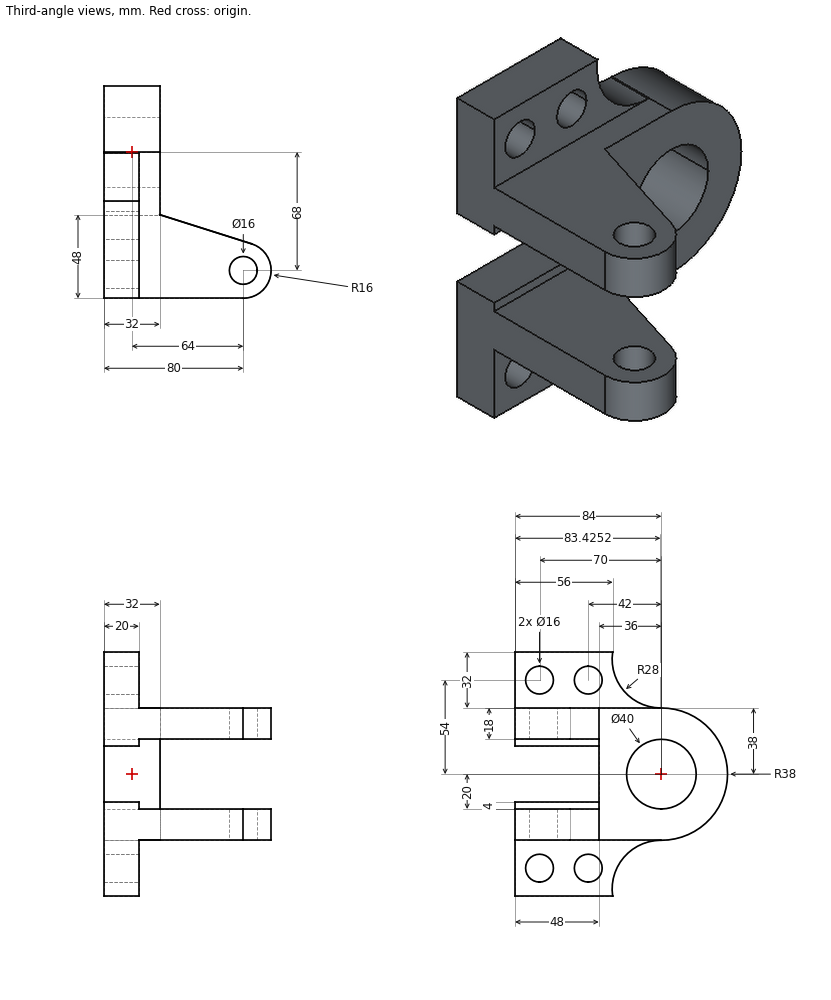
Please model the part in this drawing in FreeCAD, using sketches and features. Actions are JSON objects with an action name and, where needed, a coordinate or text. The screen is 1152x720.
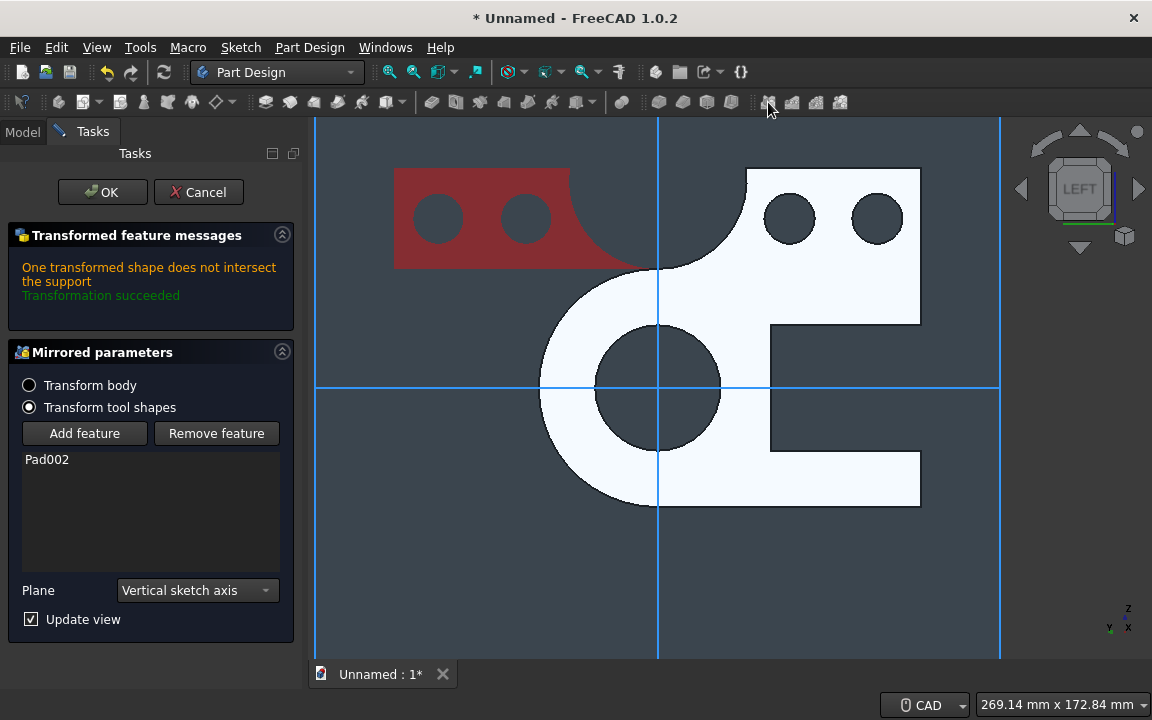
{"action": "left_click", "coordinate": [198, 590]}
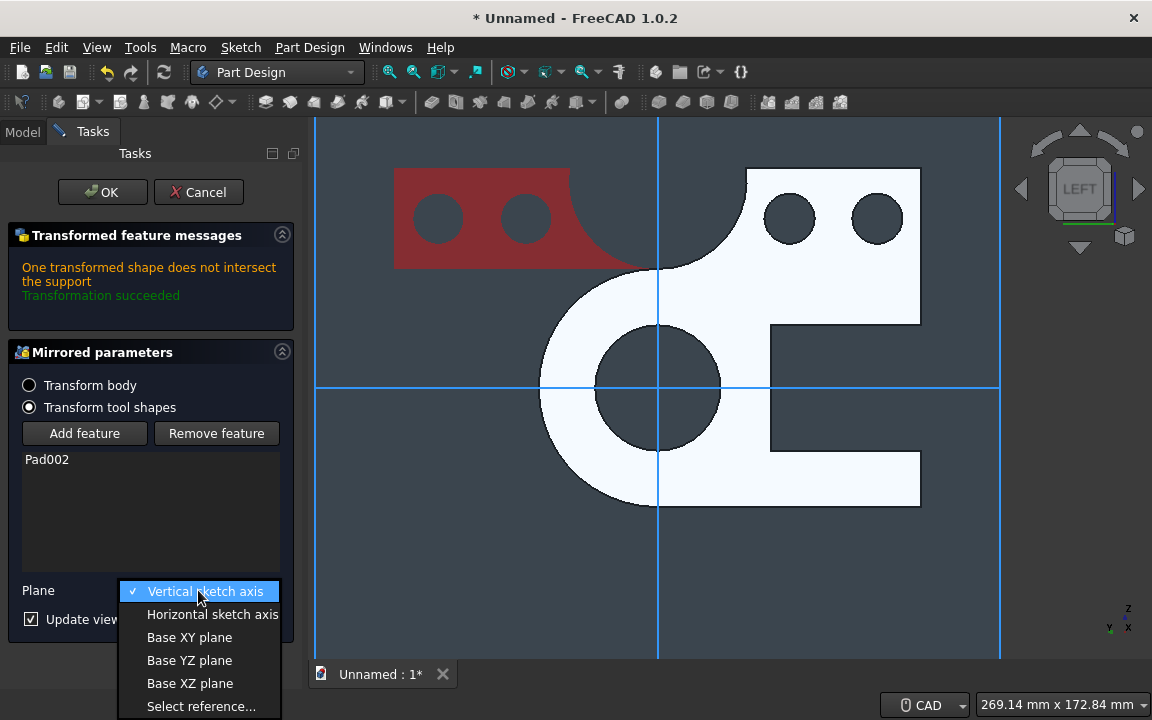
{"action": "left_click", "coordinate": [198, 638]}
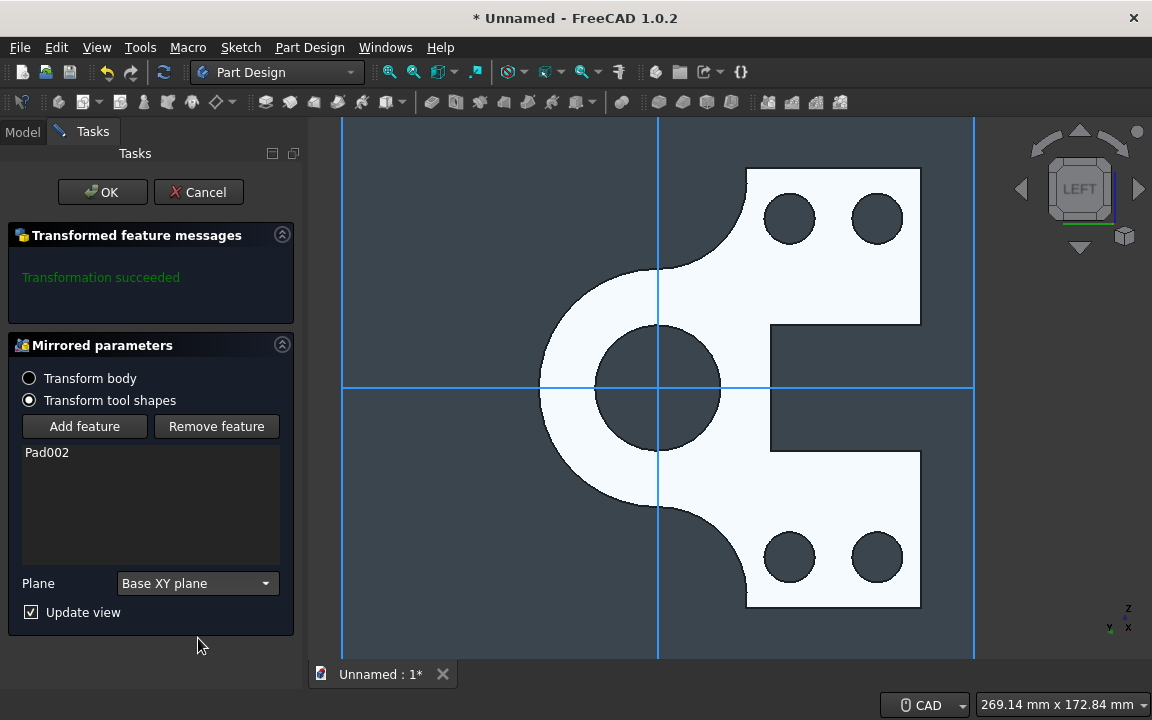
{"action": "left_click", "coordinate": [103, 192]}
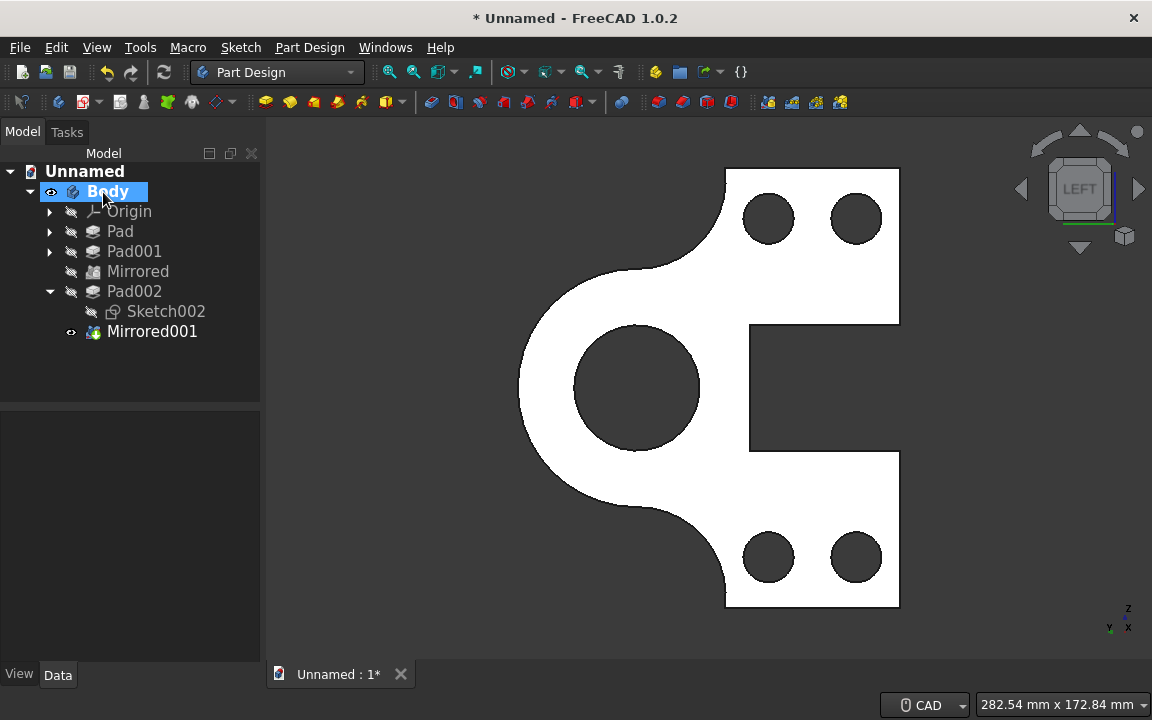
{"action": "left_click", "coordinate": [818, 512]}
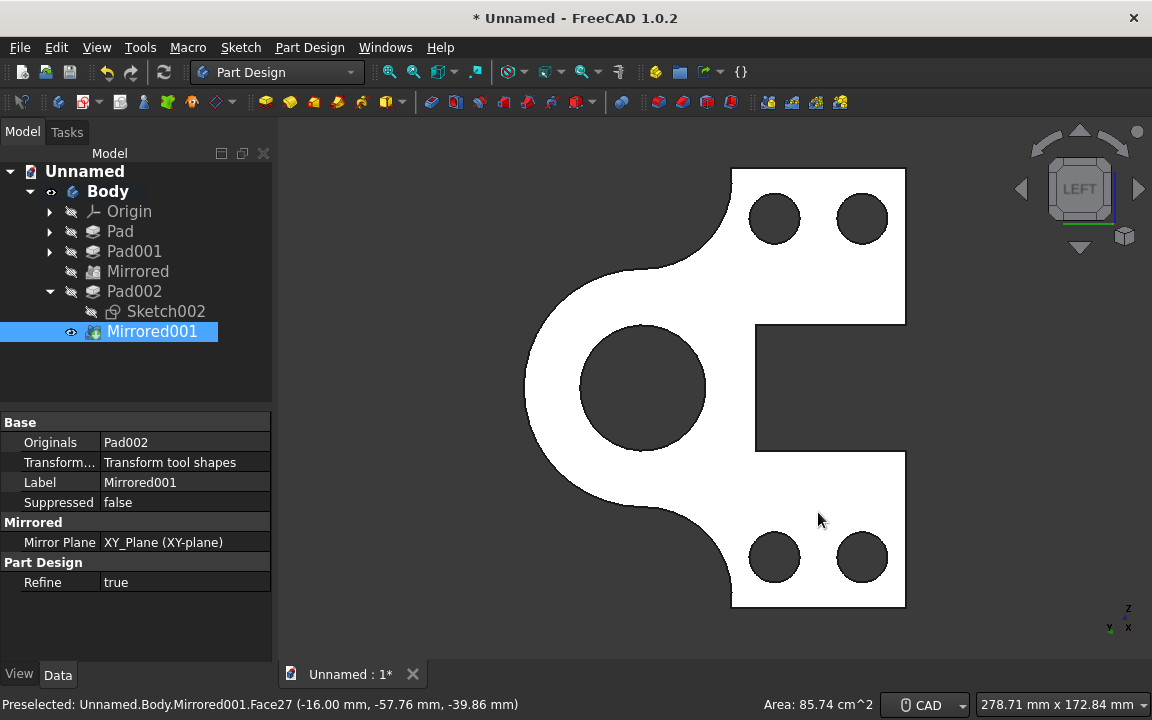
{"action": "left_click", "coordinate": [84, 102]}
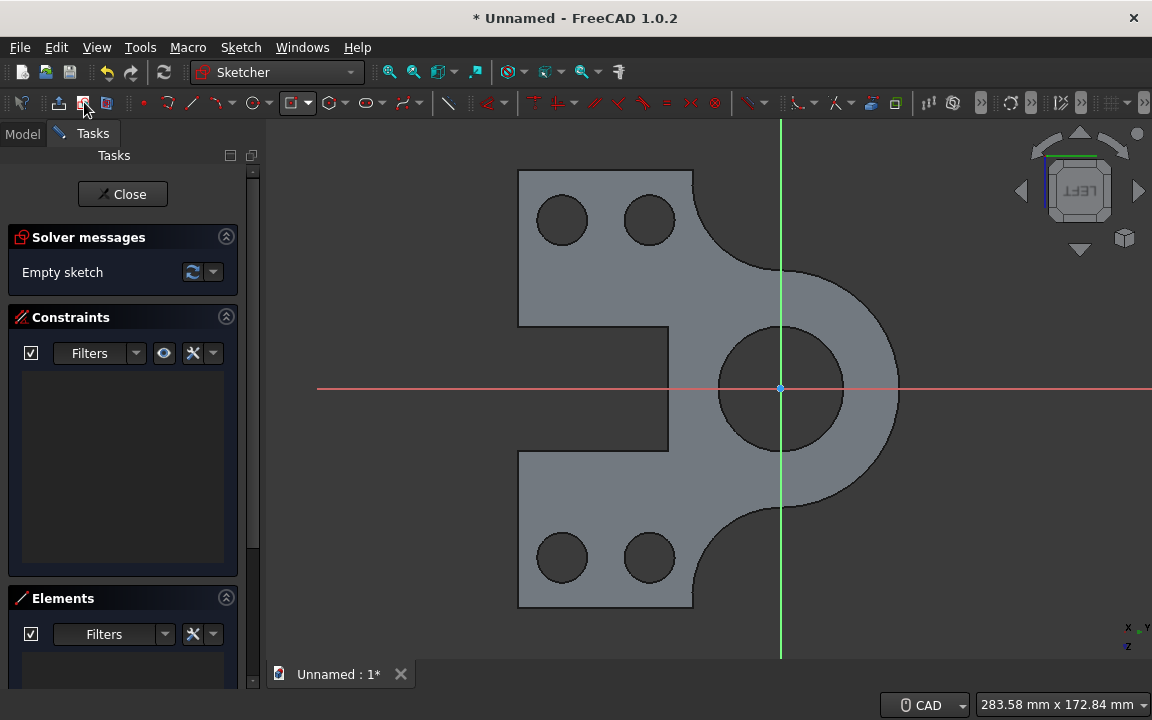
{"action": "scroll", "coordinate": [661, 320], "scroll_direction": "up", "scroll_amount": 3}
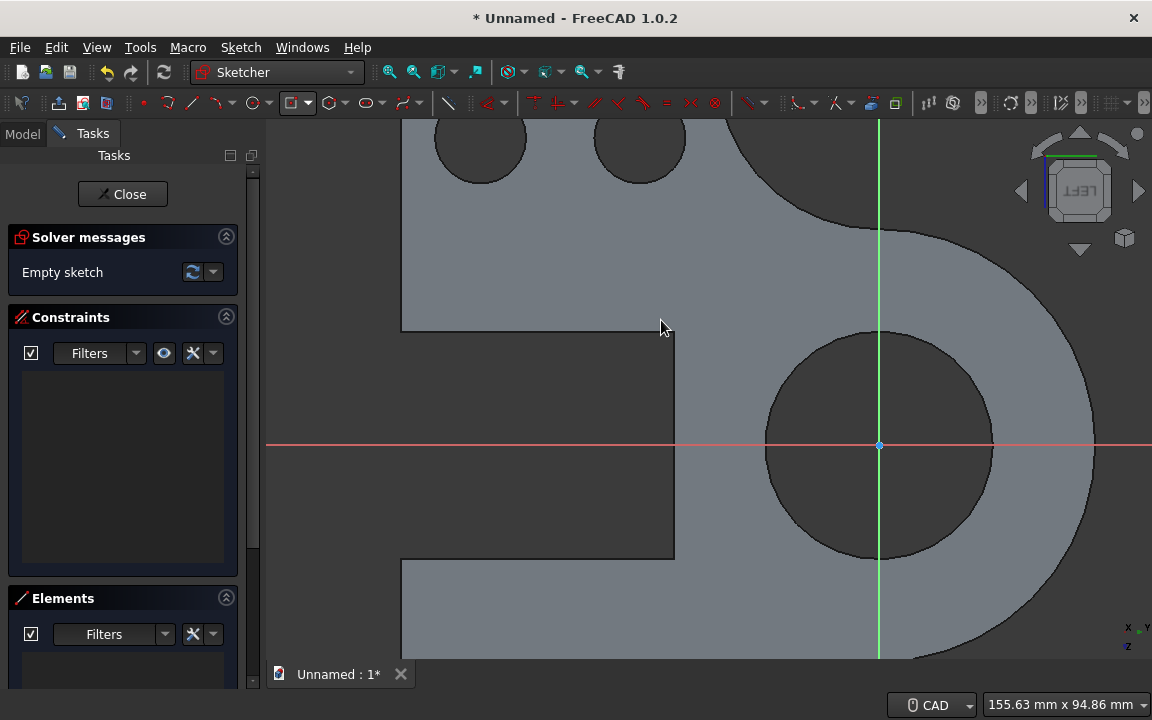
{"action": "key", "text": "g r"}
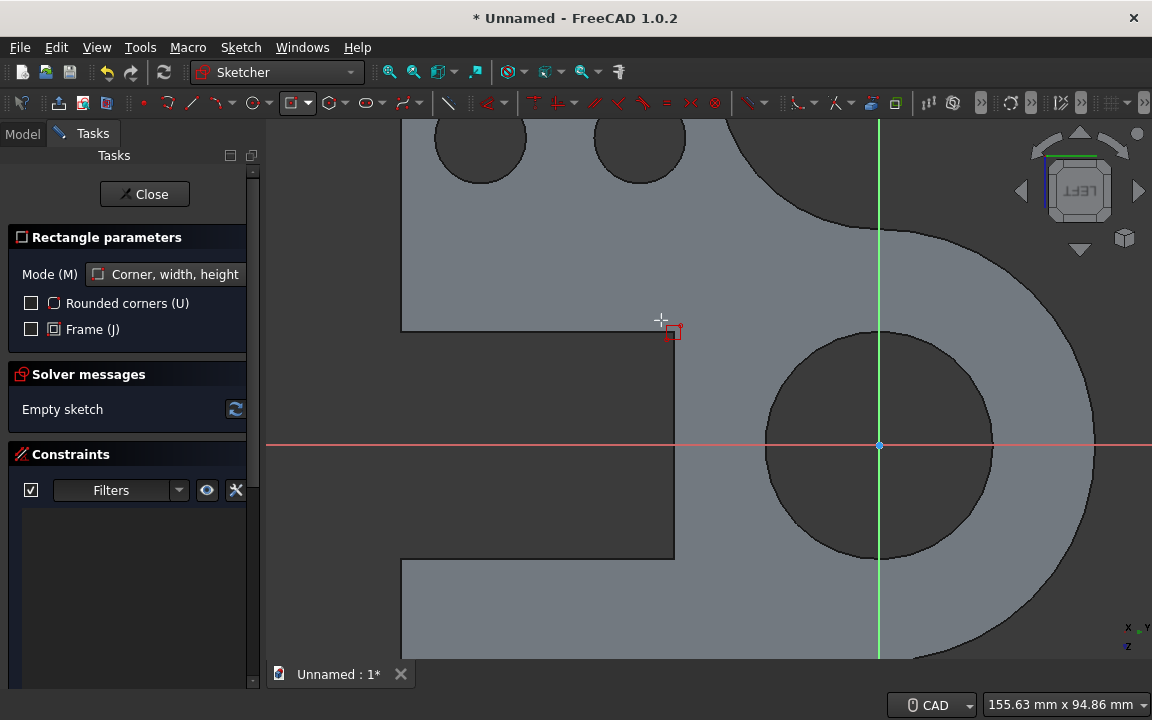
{"action": "left_click", "coordinate": [401, 332]}
{"action": "left_click", "coordinate": [674, 354]}
{"action": "key", "text": "Escape"}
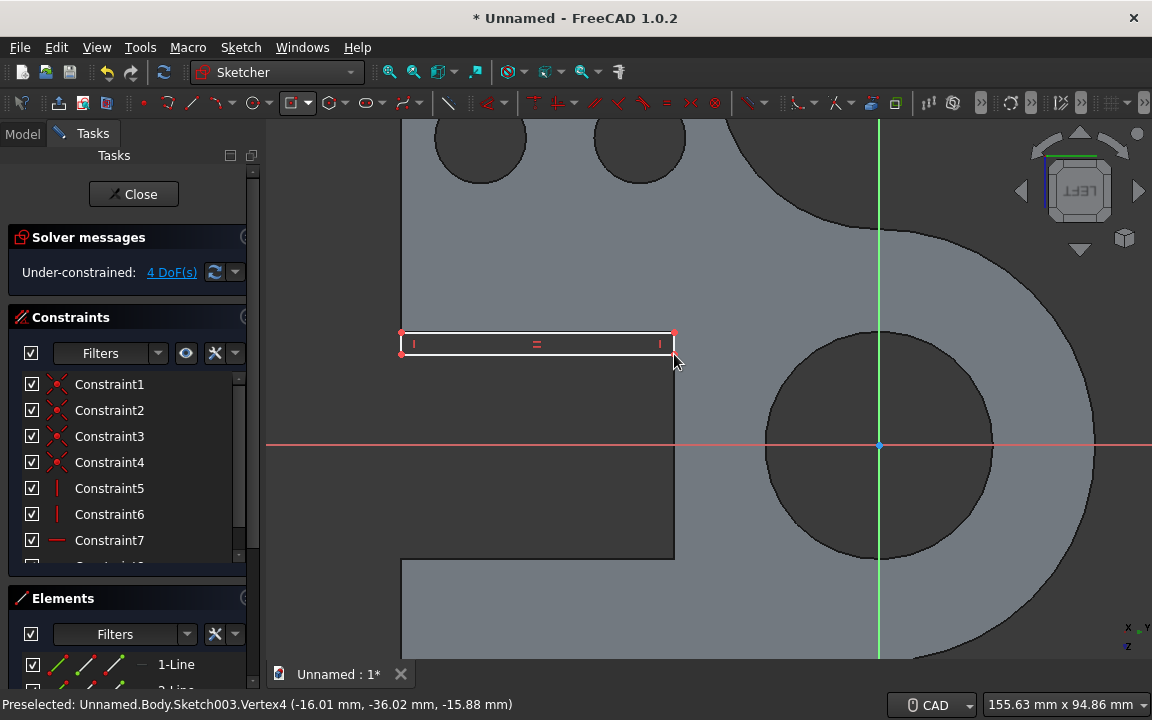
{"action": "left_click", "coordinate": [488, 104]}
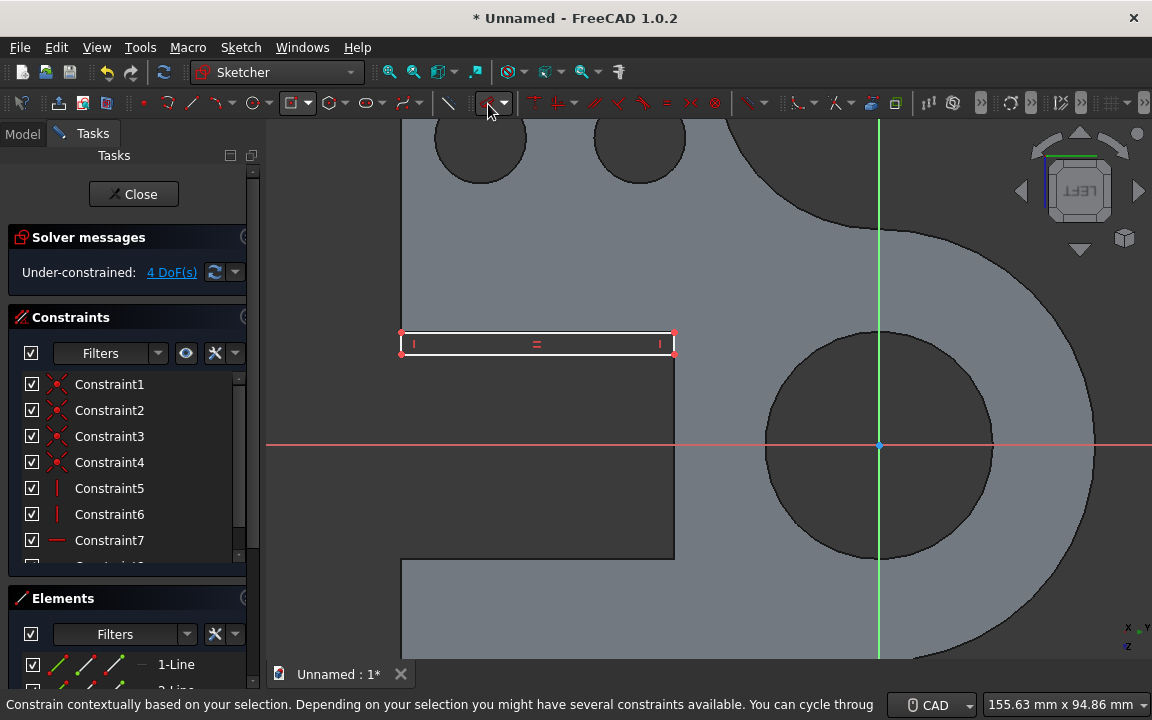
{"action": "scroll", "coordinate": [401, 344], "scroll_direction": "up", "scroll_amount": 3}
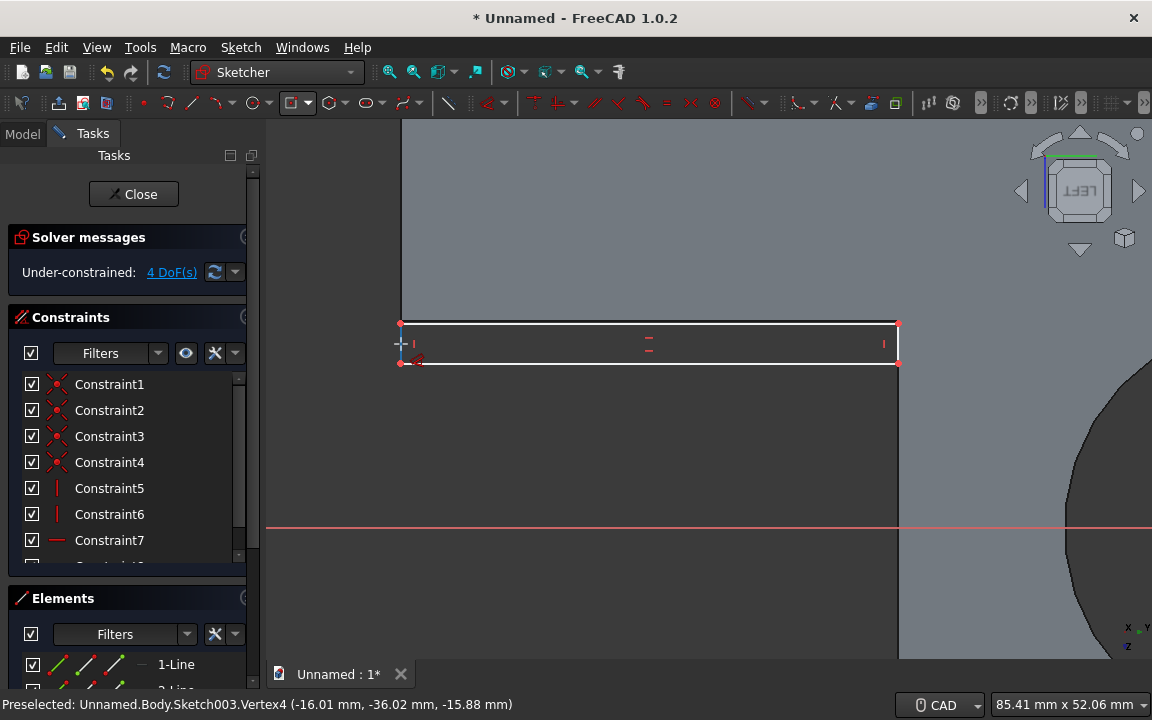
{"action": "left_click", "coordinate": [401, 344]}
{"action": "left_click", "coordinate": [367, 344]}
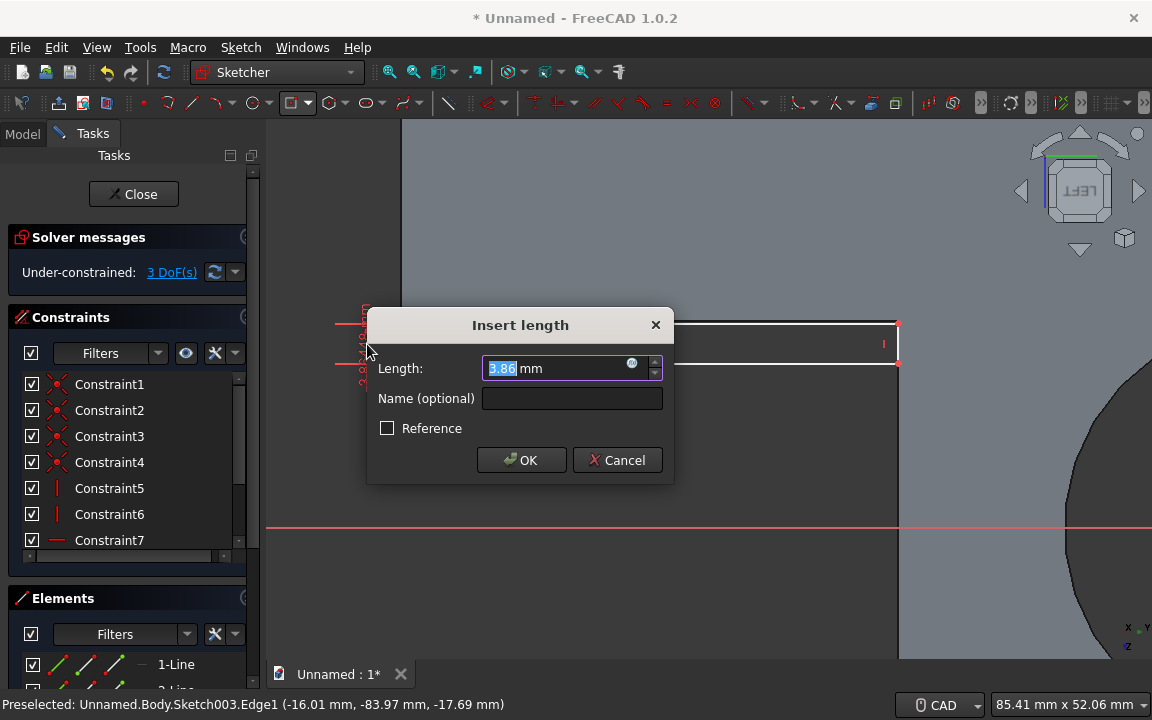
{"action": "type", "text": "4"}
{"action": "key", "text": "Return"}